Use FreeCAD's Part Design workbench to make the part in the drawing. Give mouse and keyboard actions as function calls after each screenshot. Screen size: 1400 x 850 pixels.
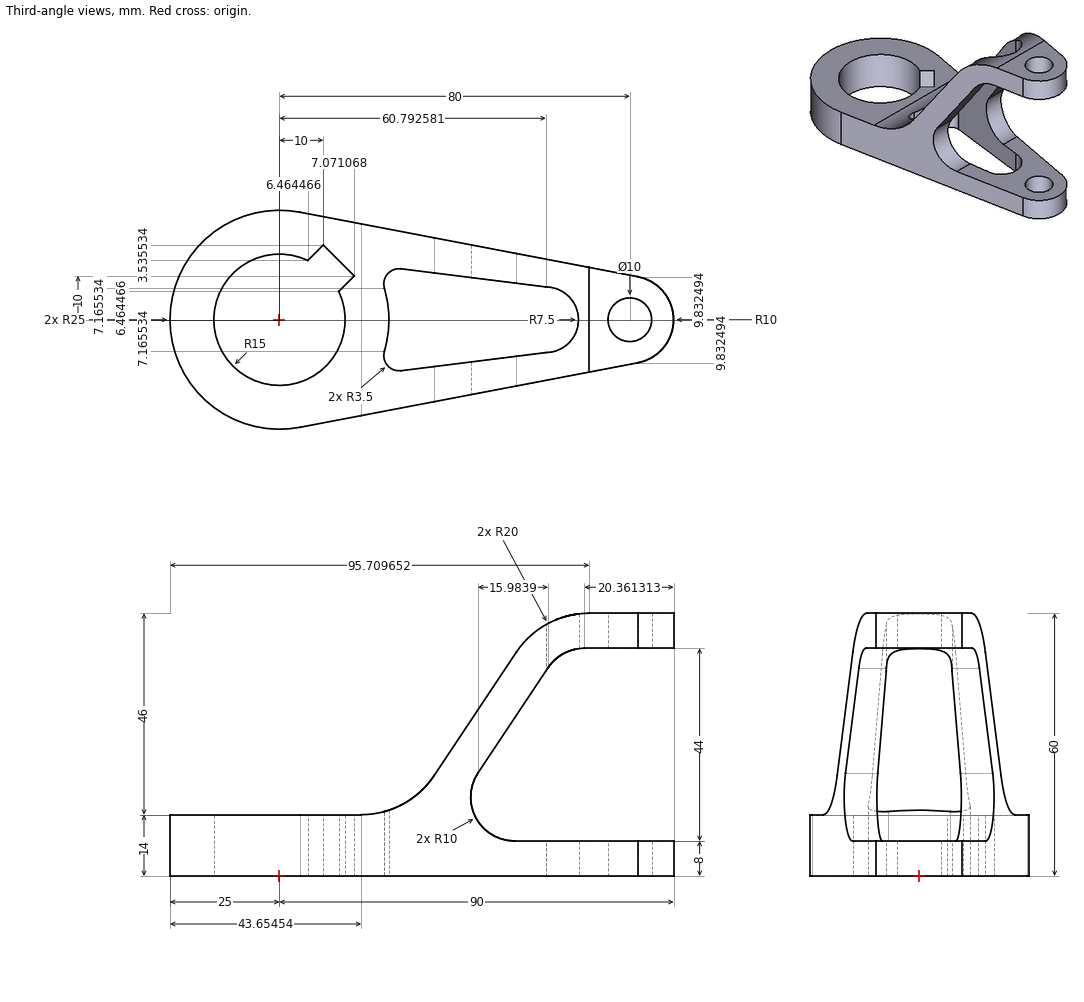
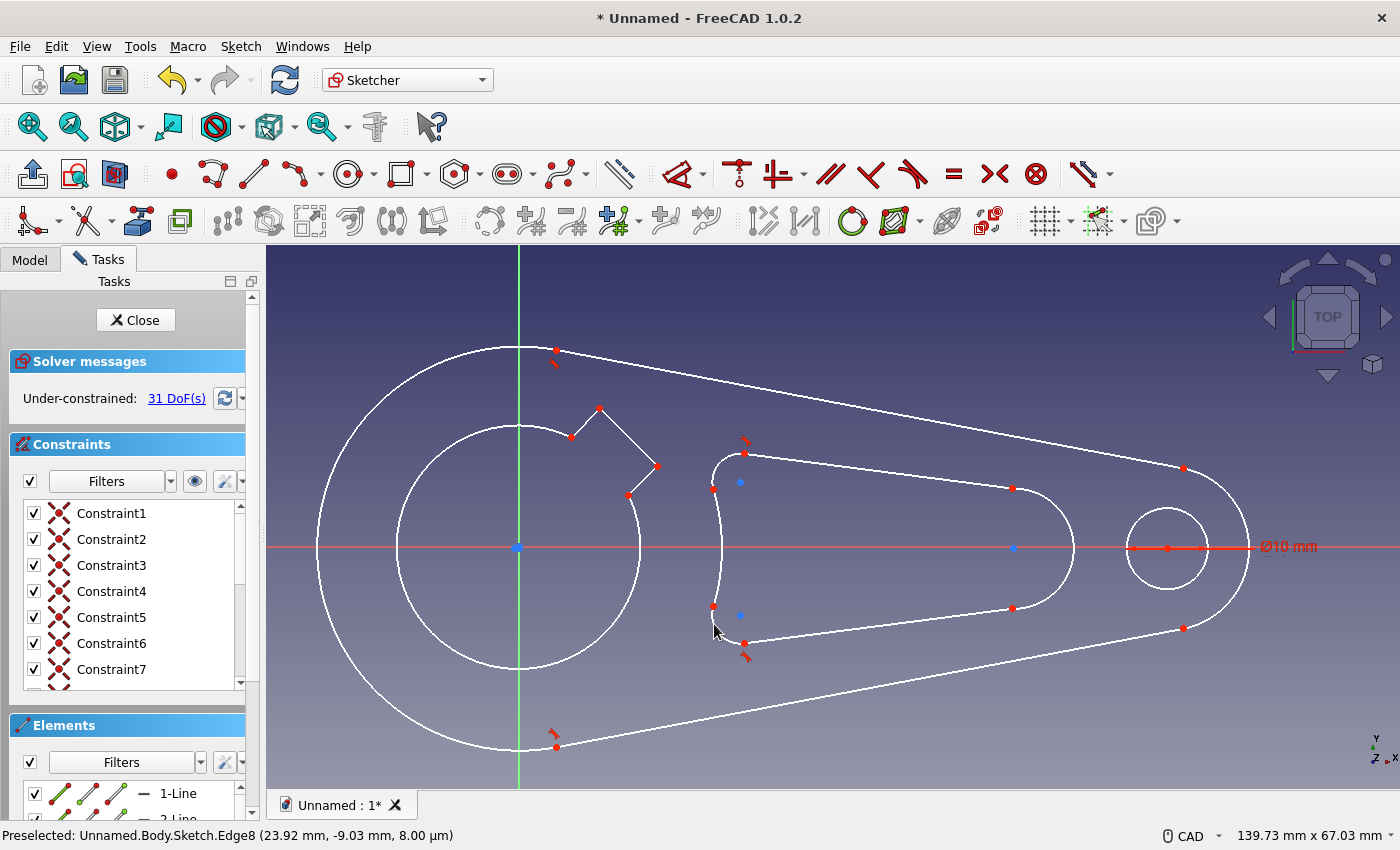
click(714, 624)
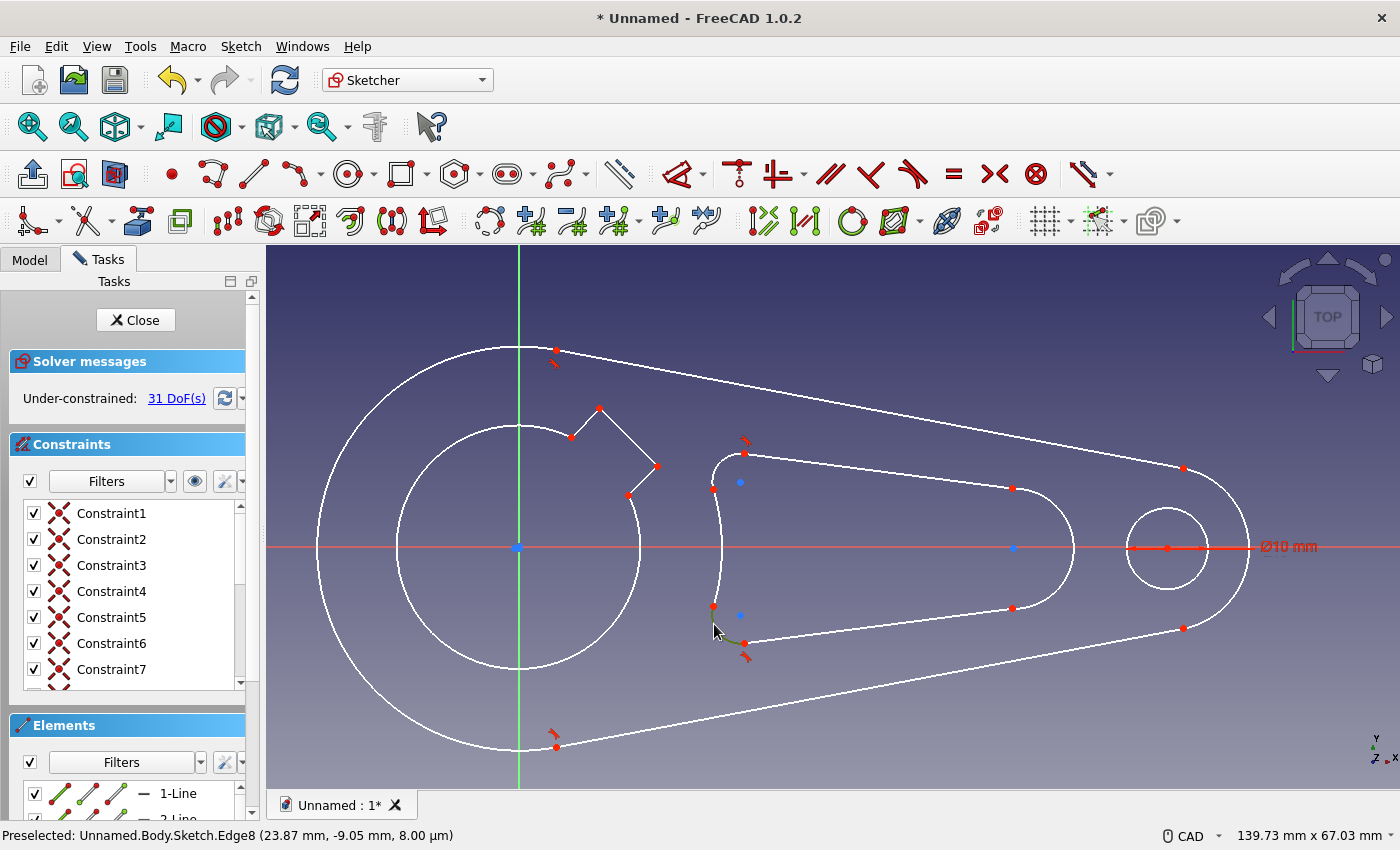
click(721, 572)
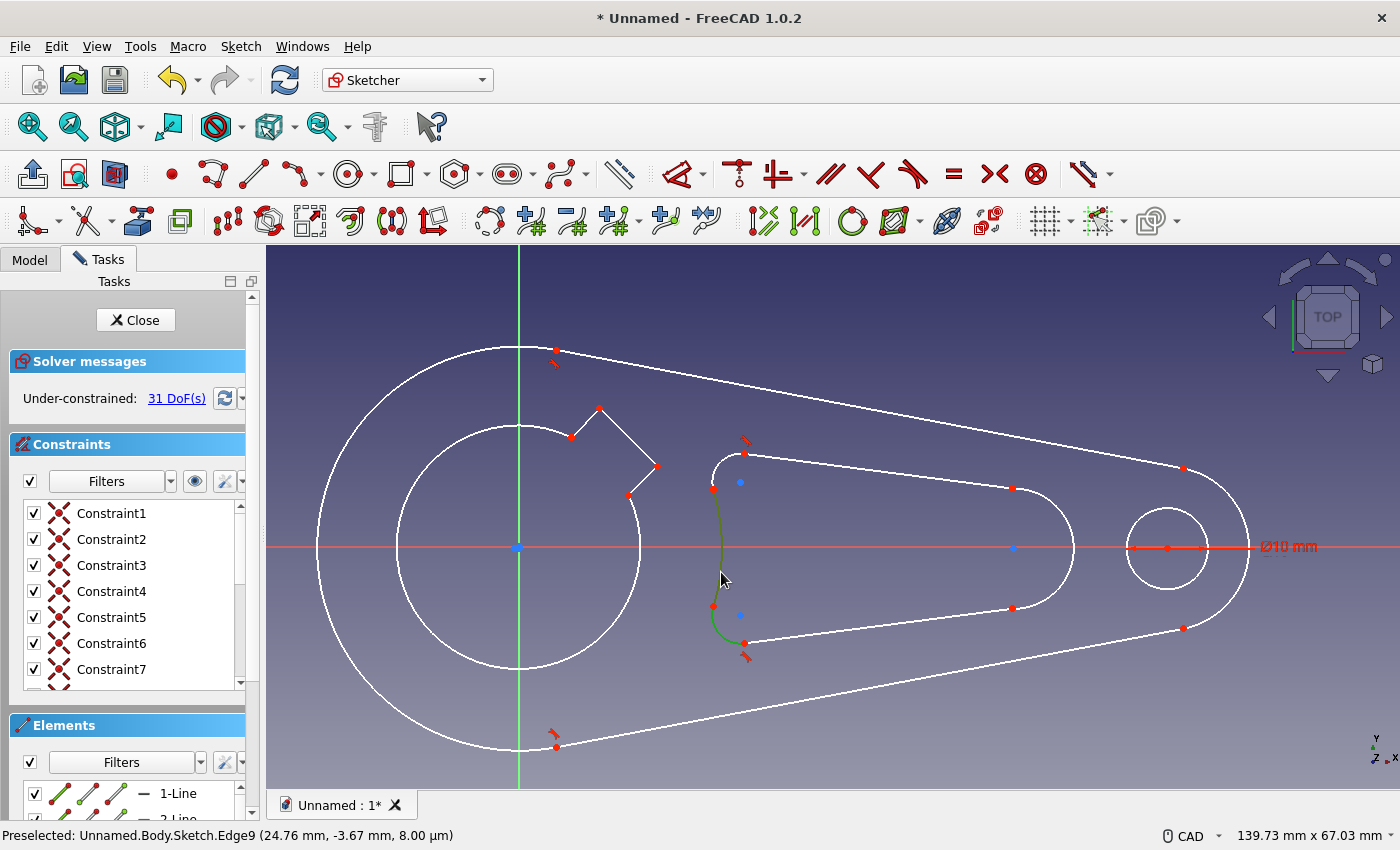
click(913, 174)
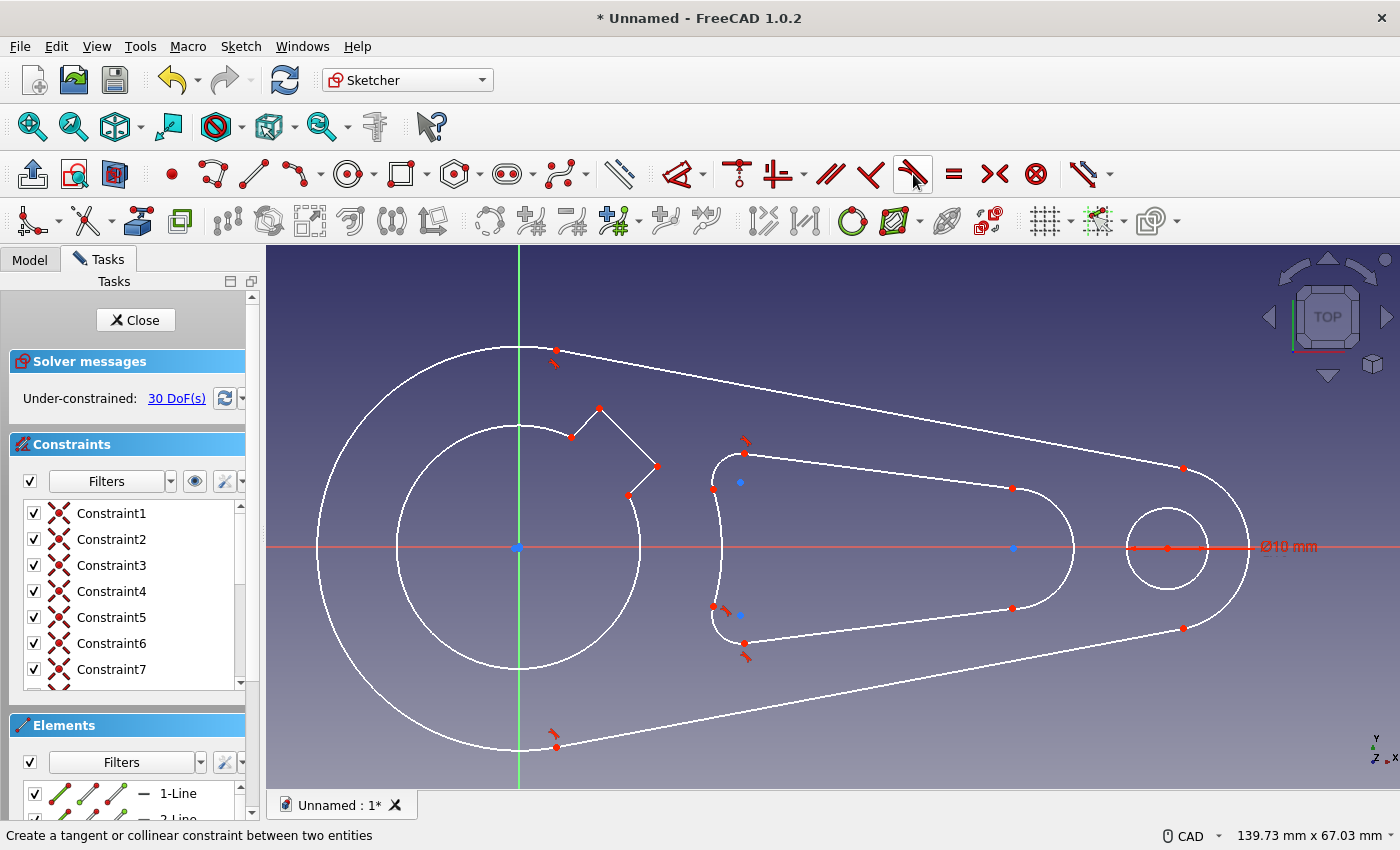
click(720, 572)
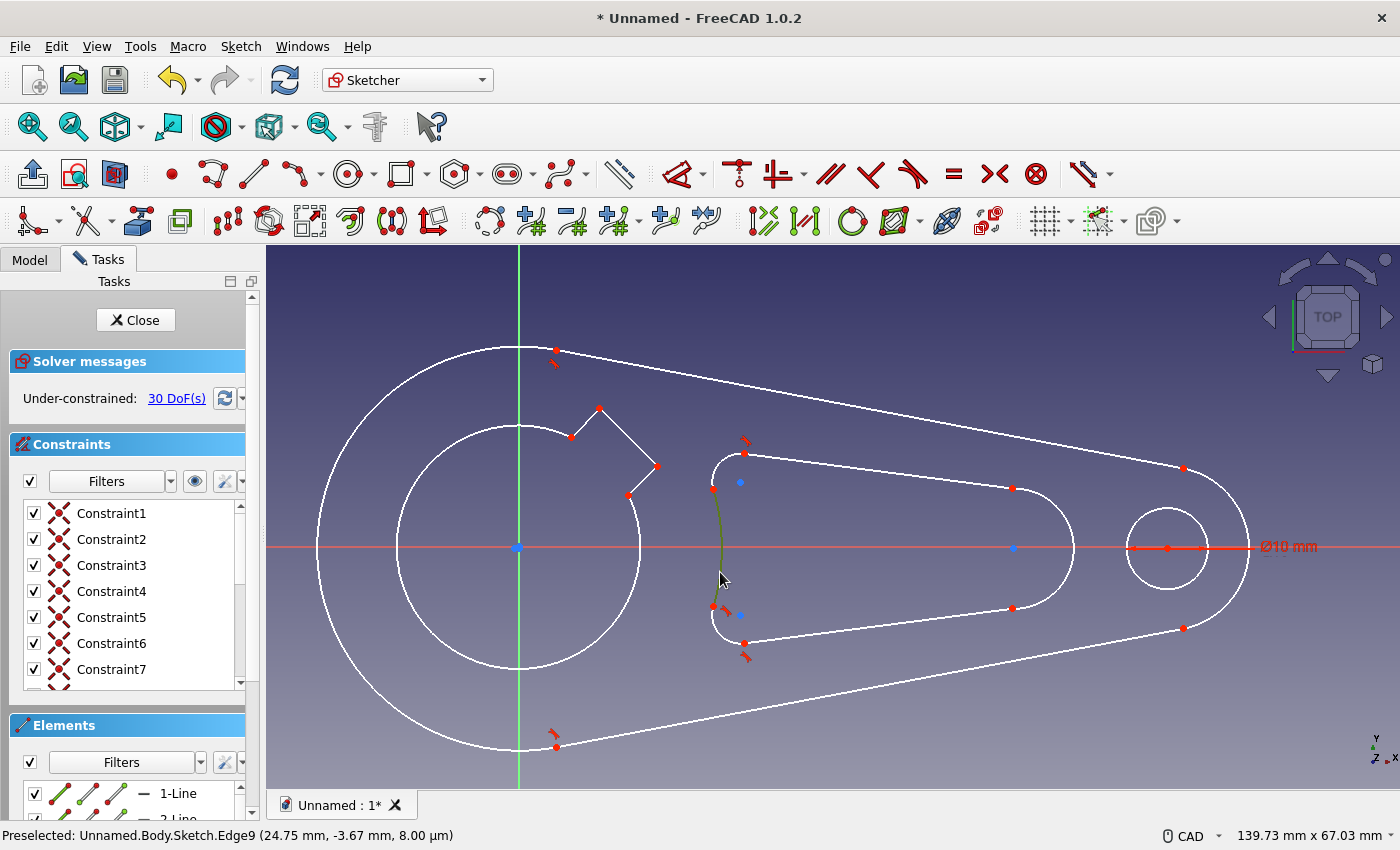
click(728, 457)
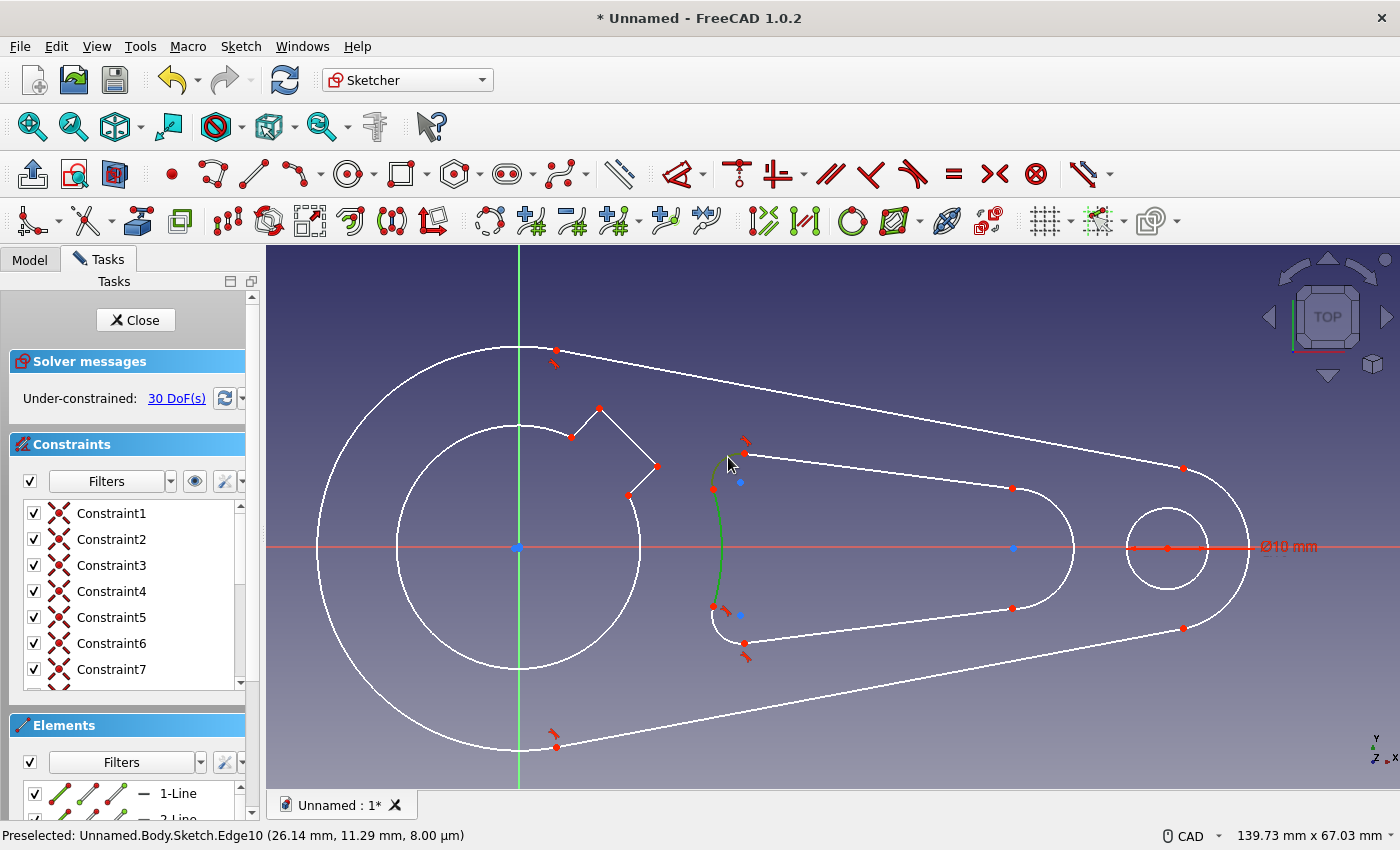
click(913, 174)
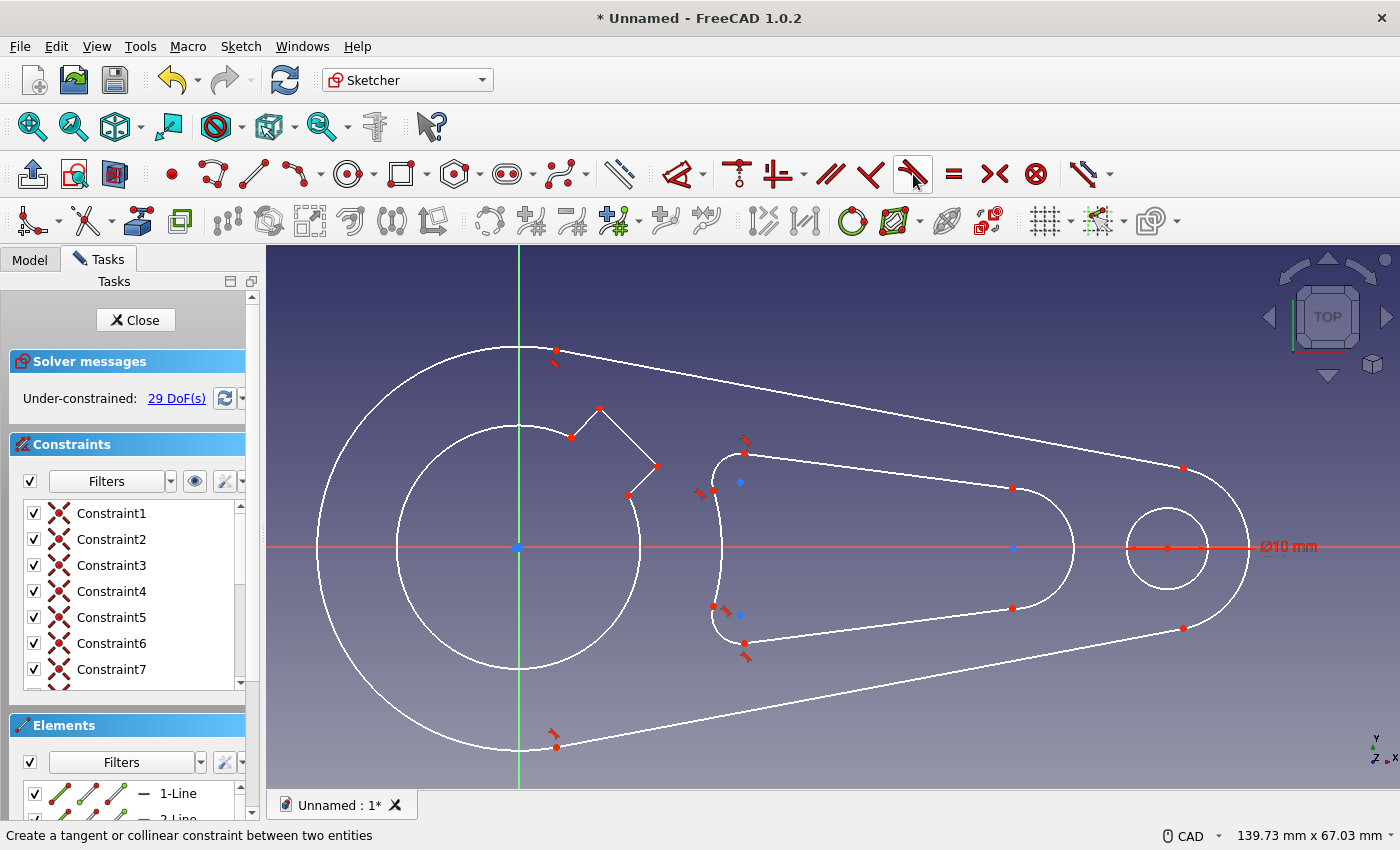
click(365, 418)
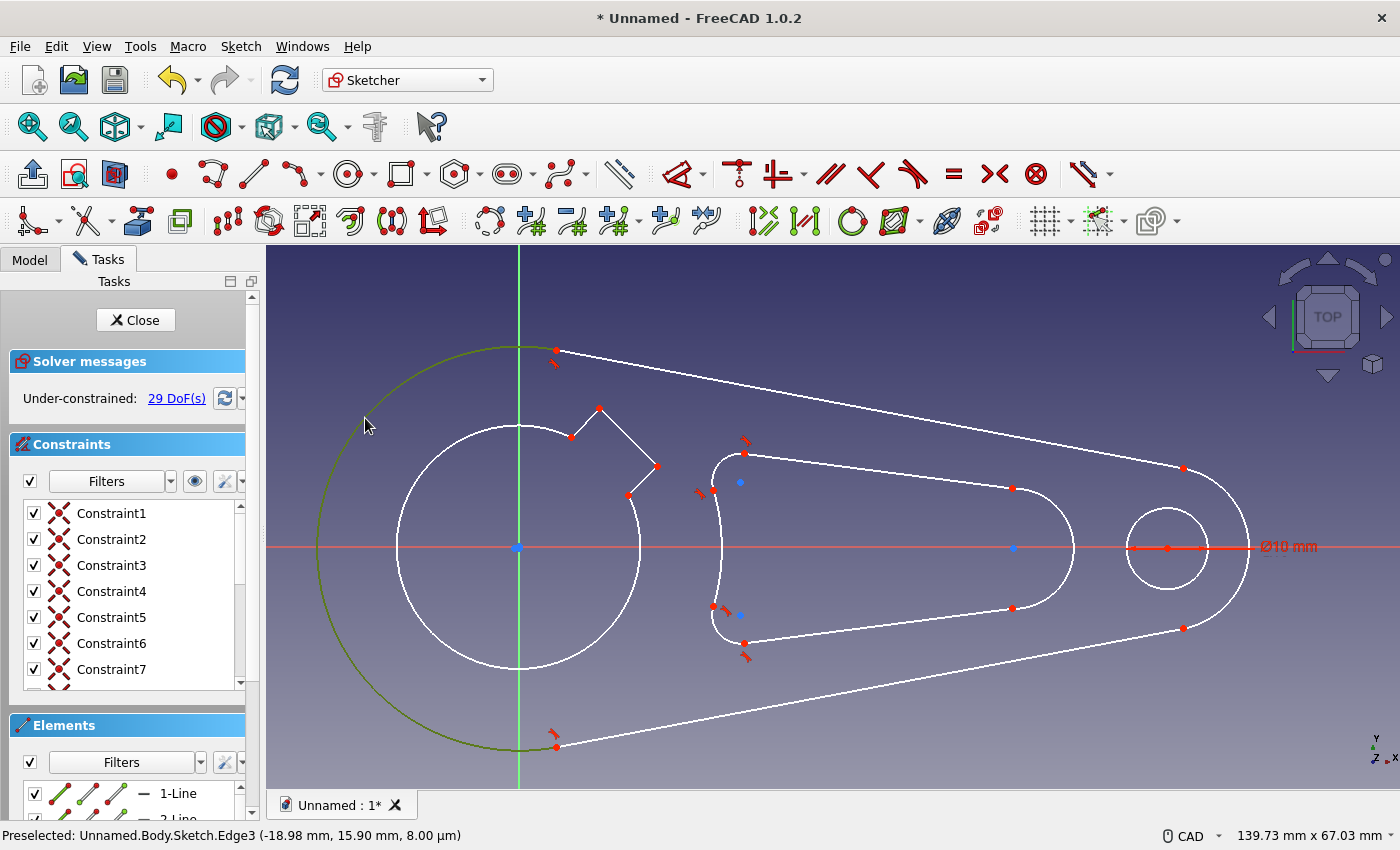
click(720, 572)